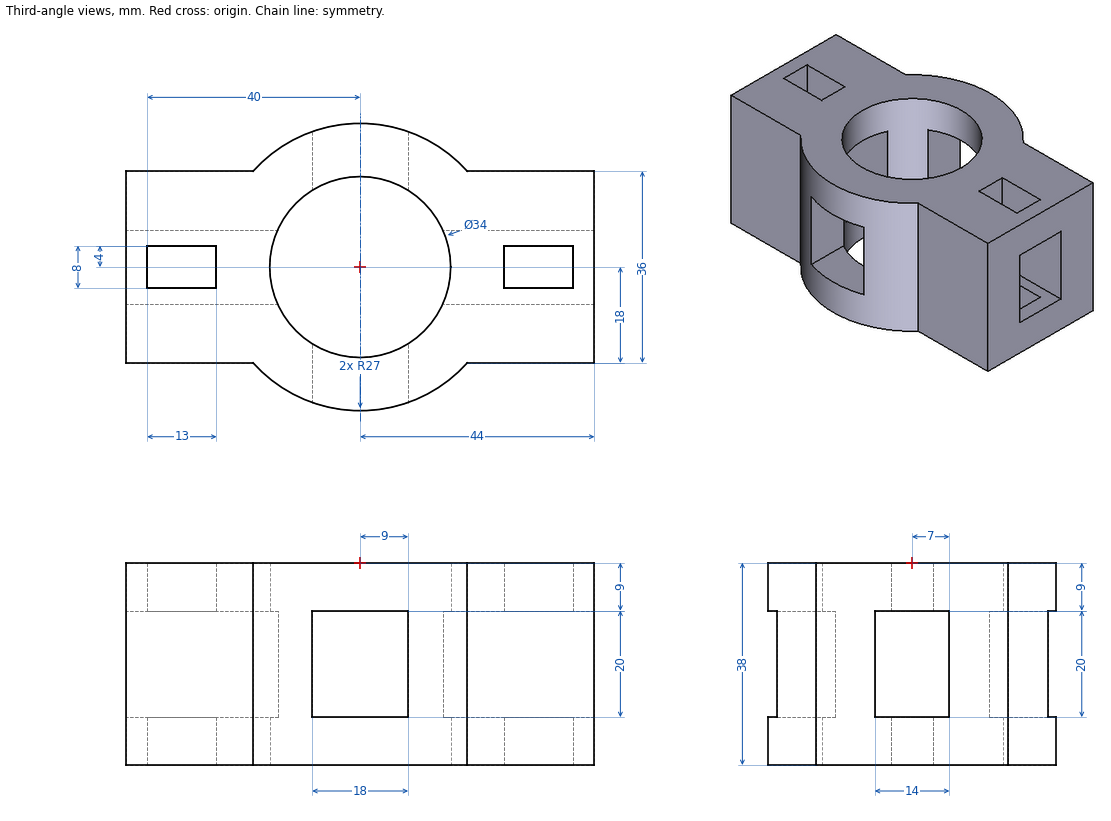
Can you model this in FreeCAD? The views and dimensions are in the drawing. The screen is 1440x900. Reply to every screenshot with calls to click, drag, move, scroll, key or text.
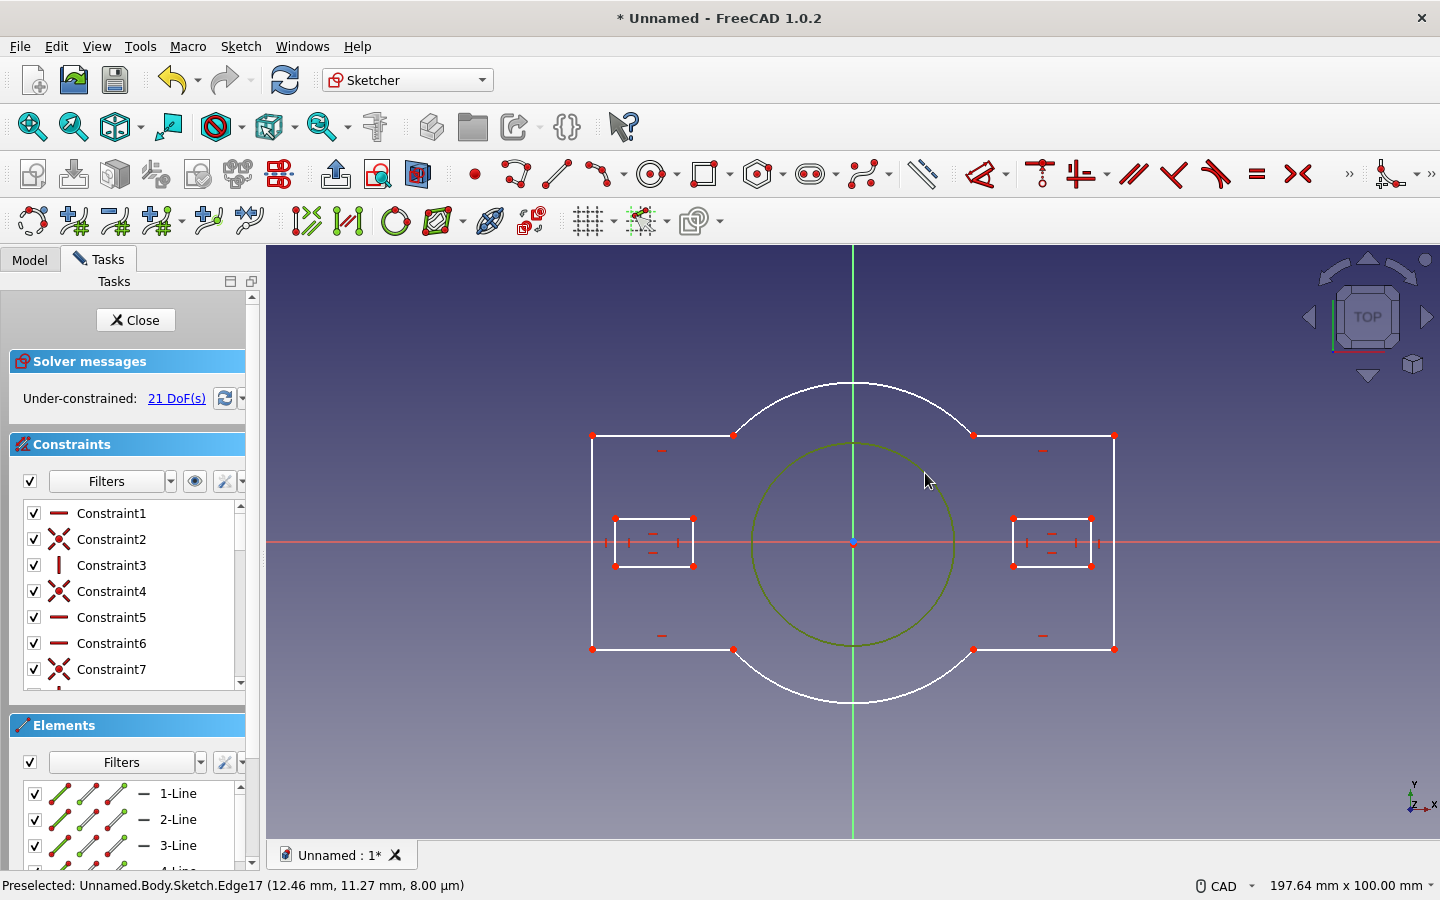
click(800, 694)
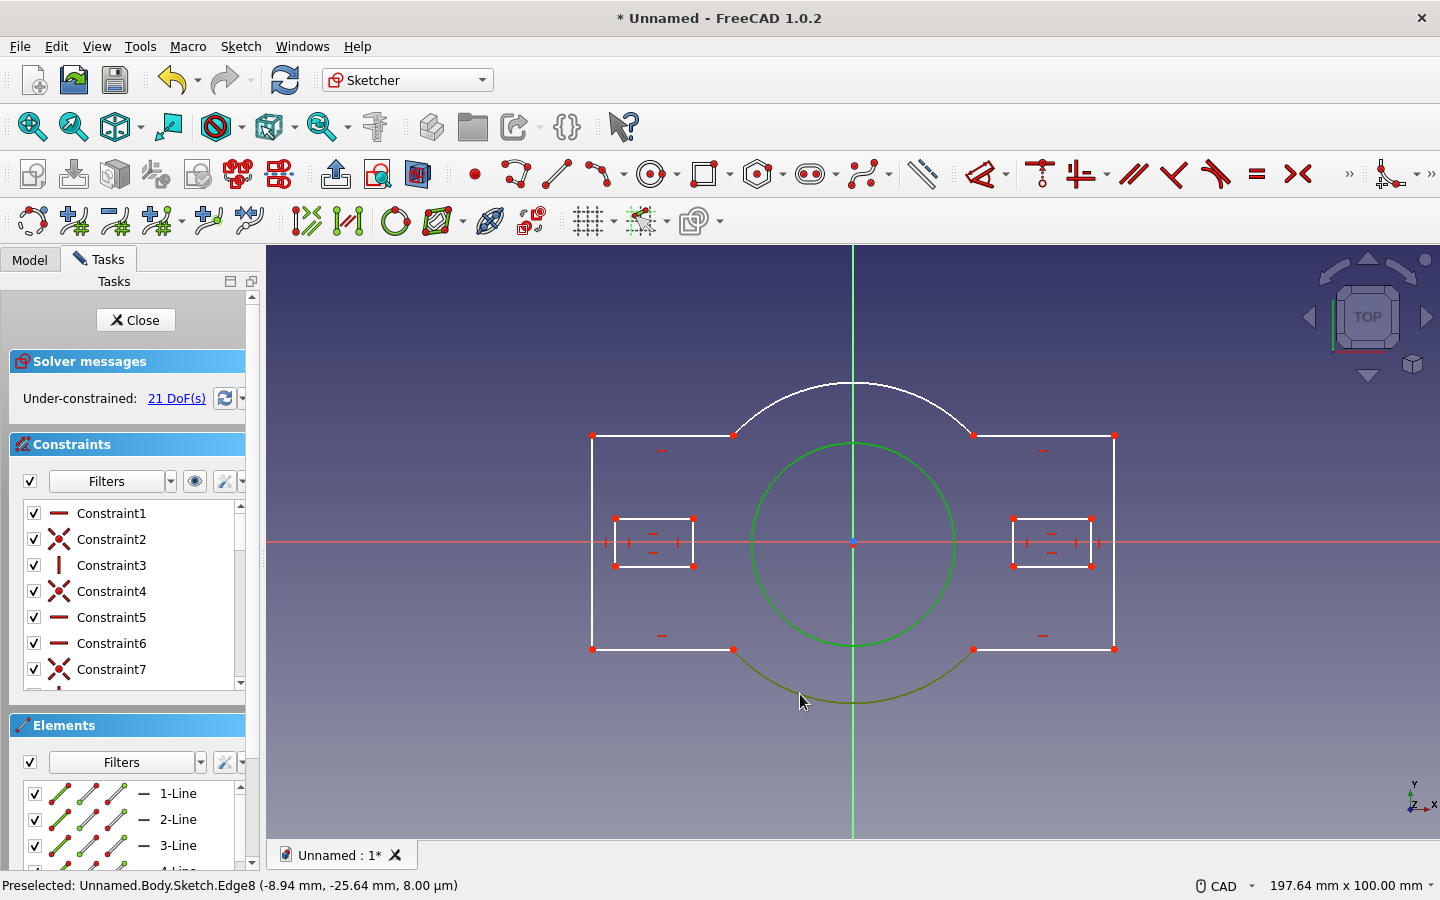
click(1040, 174)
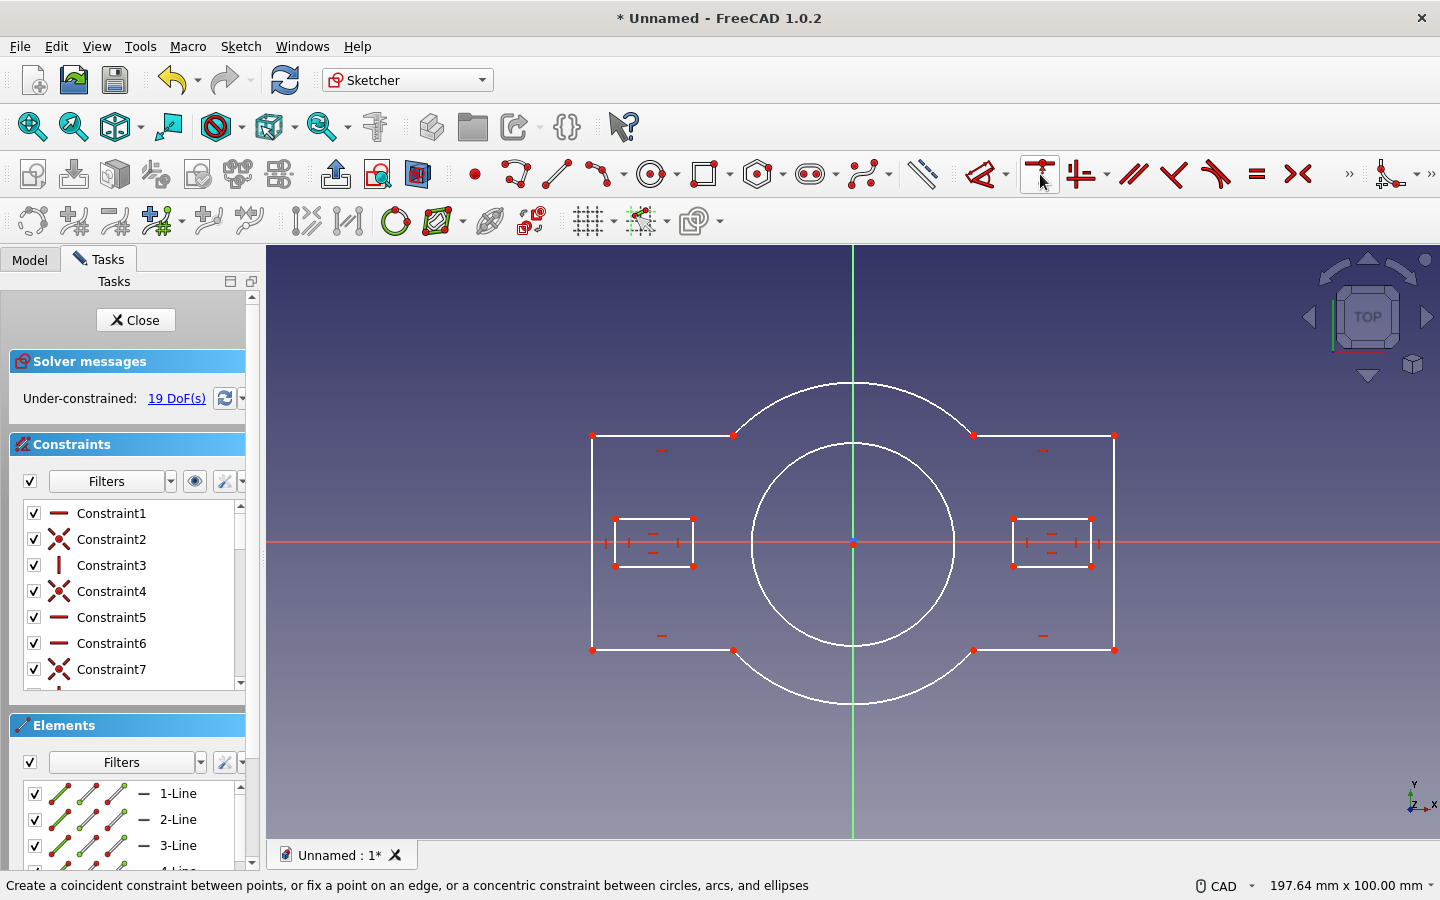
drag(843, 532, 863, 555)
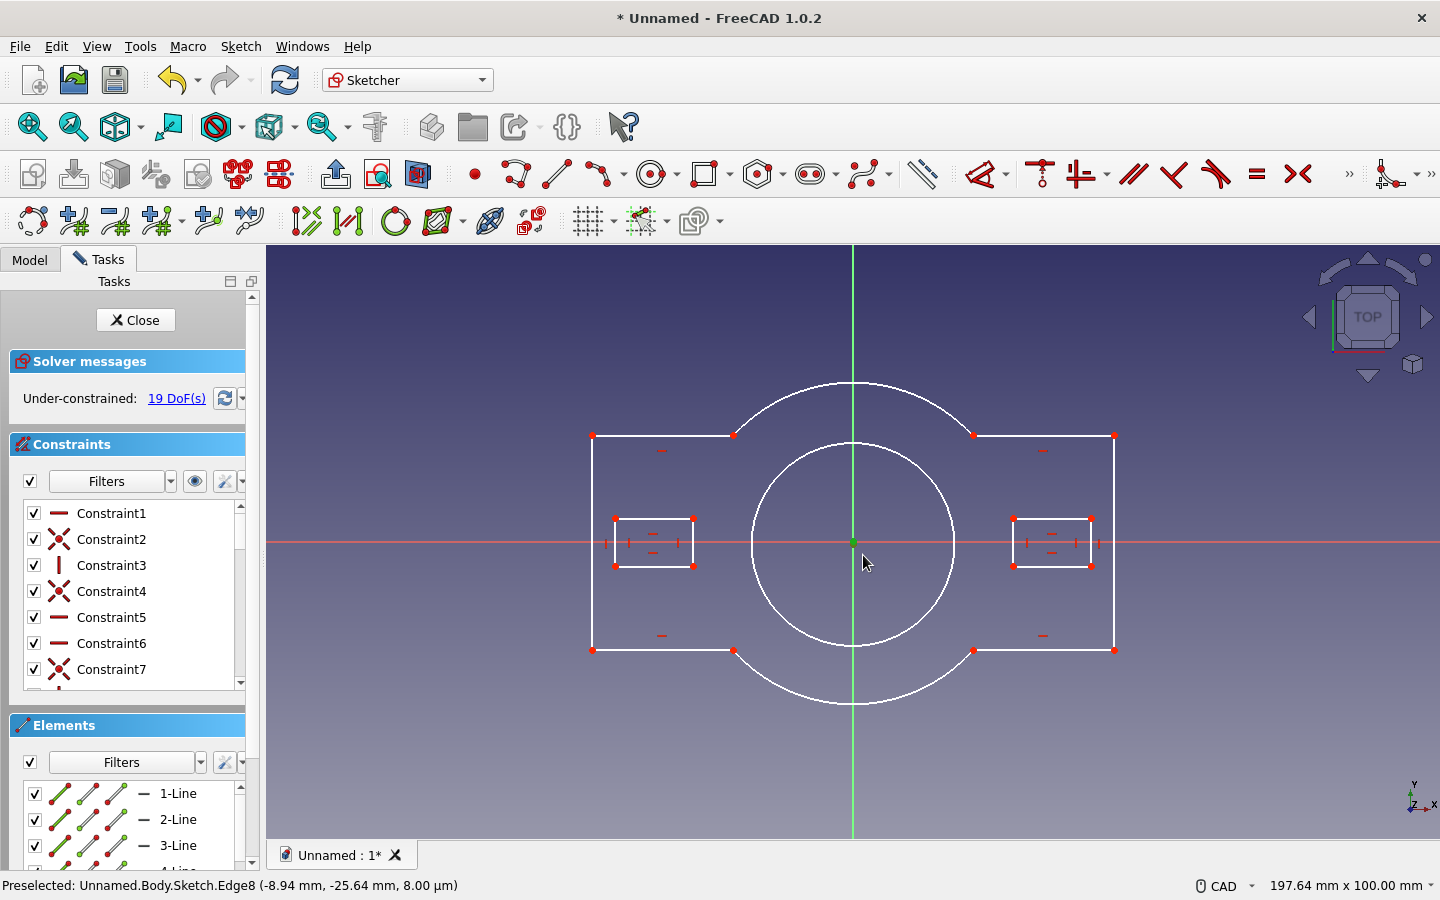
key(c)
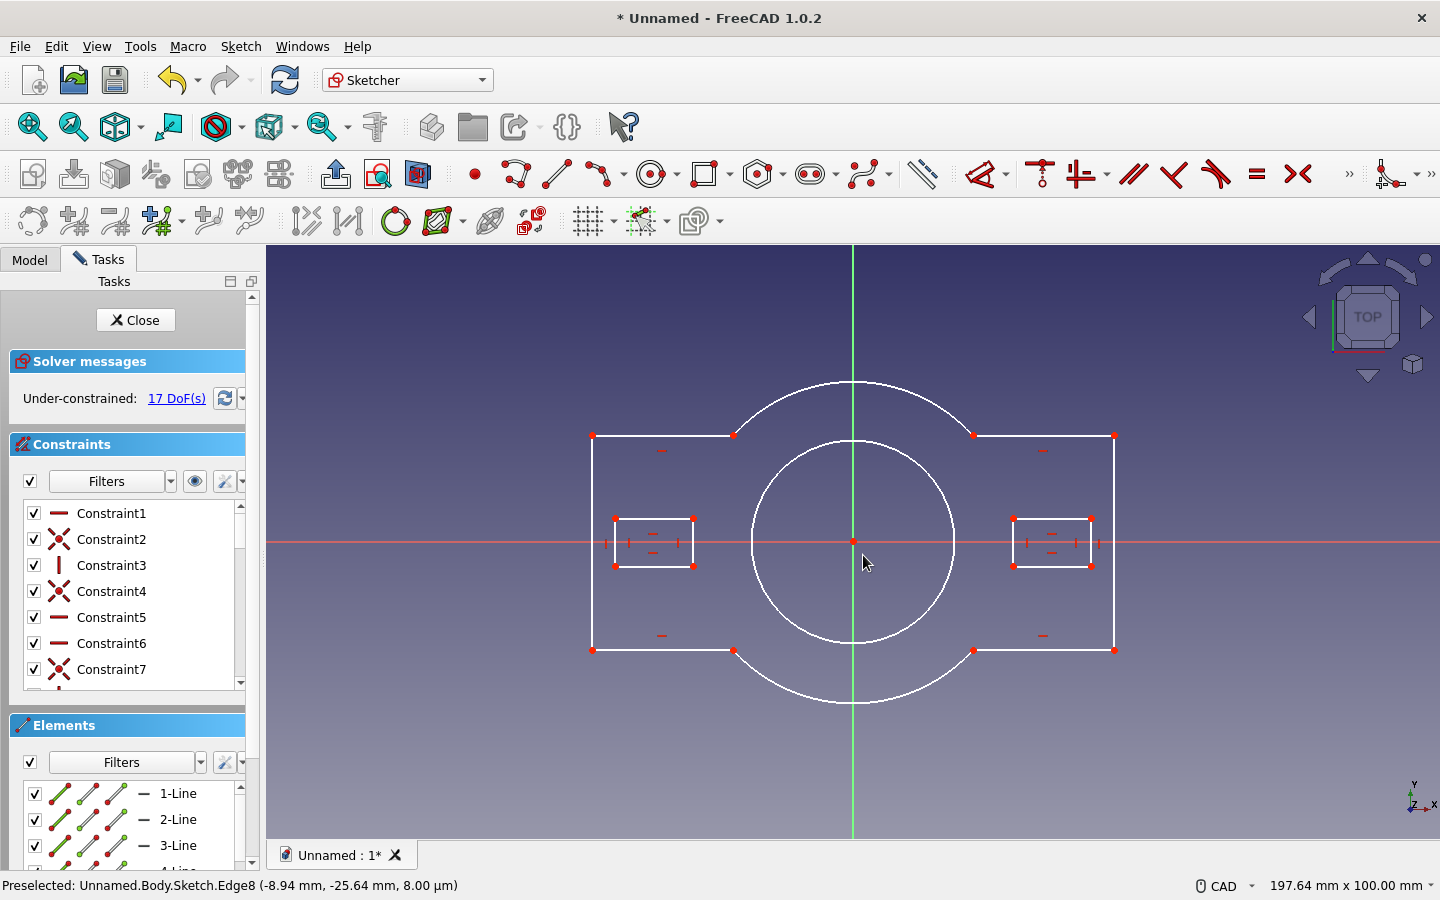
click(906, 391)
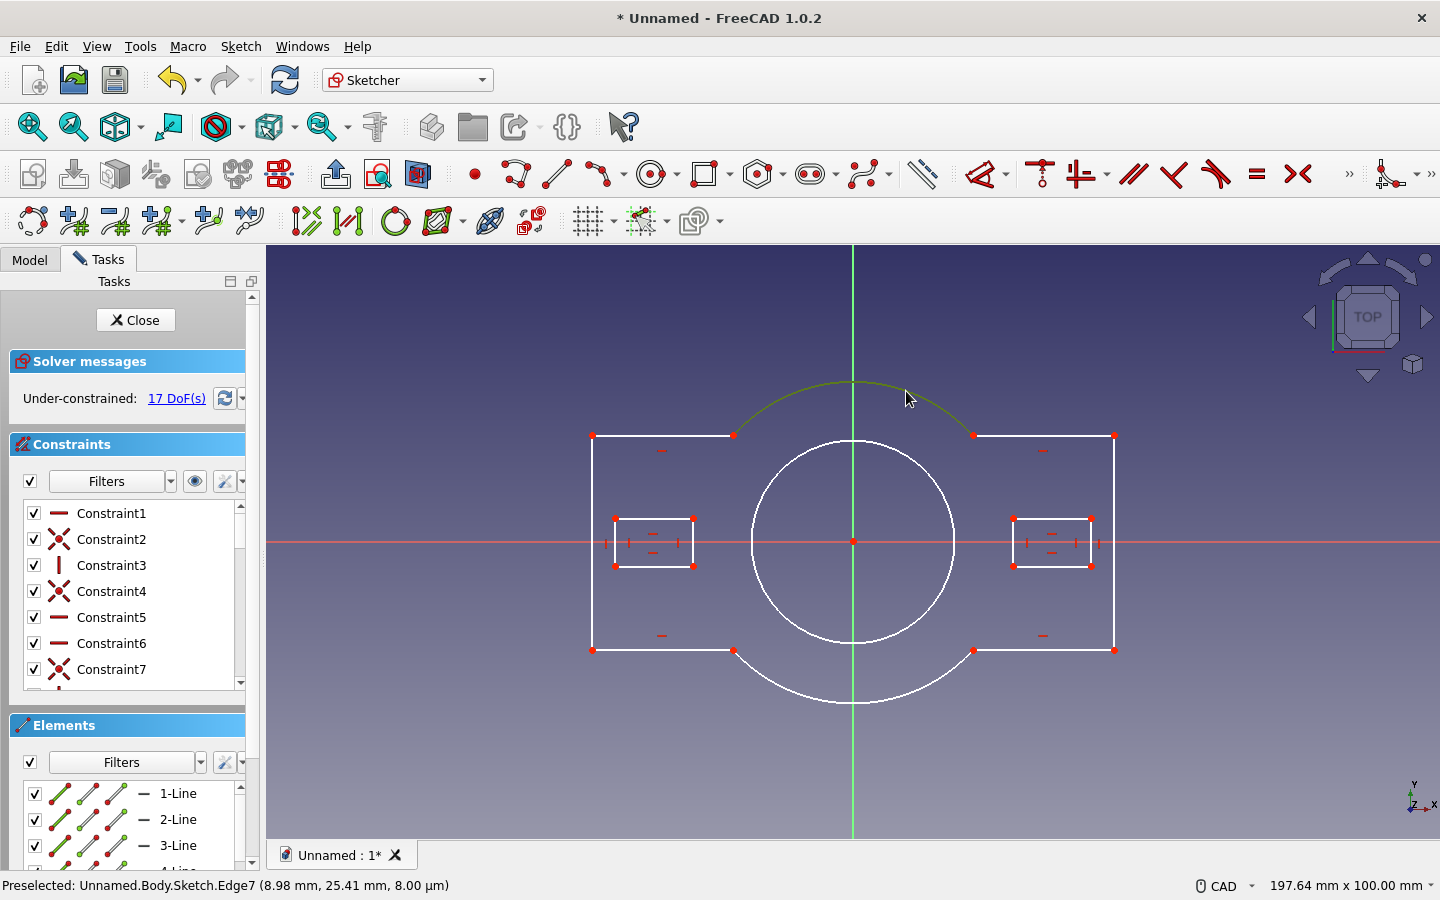
click(800, 694)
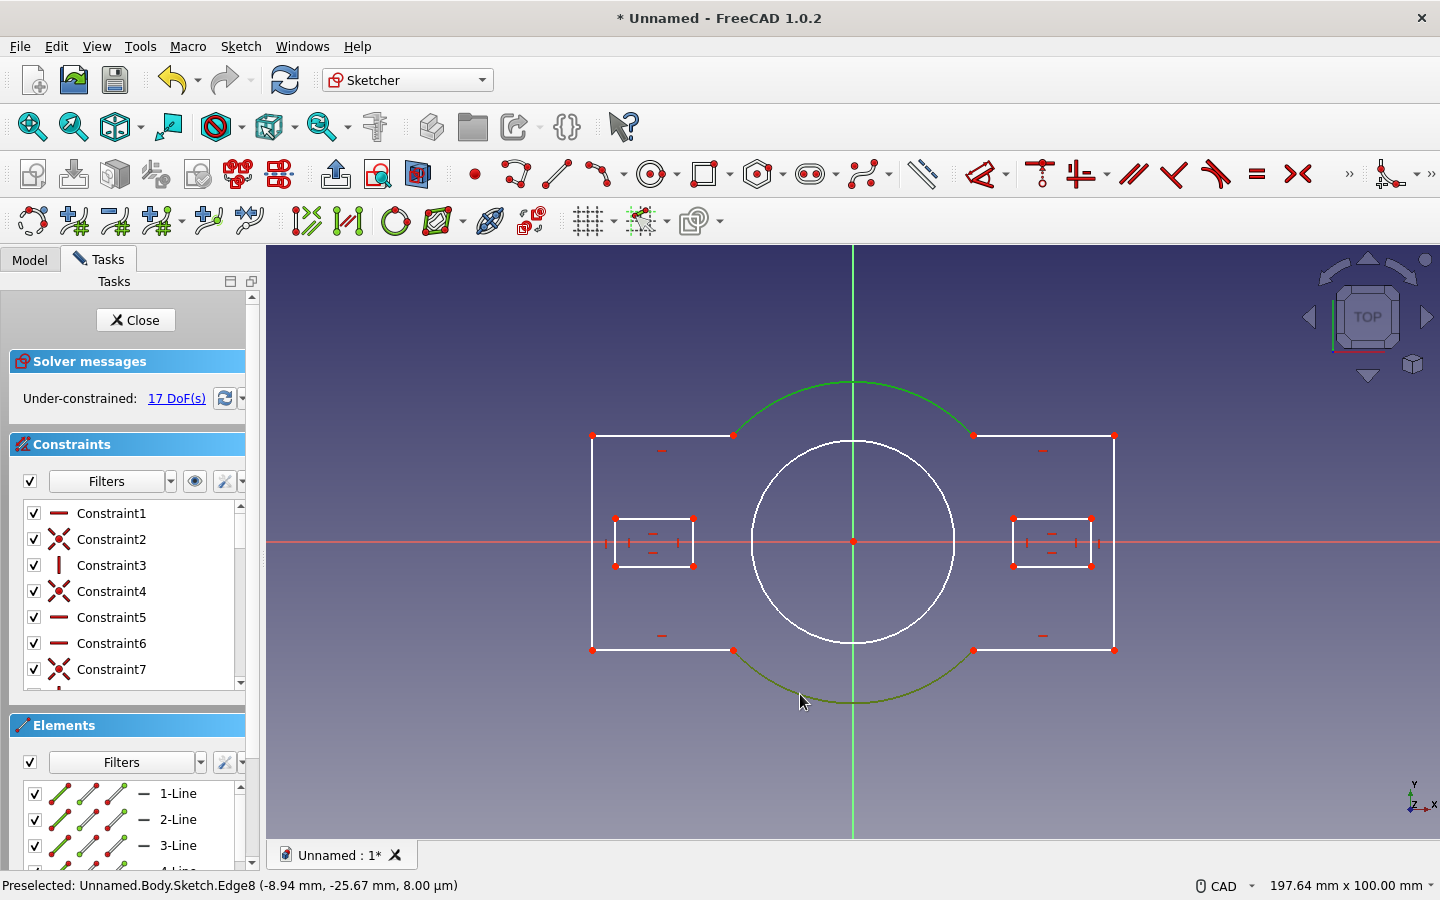
click(1257, 174)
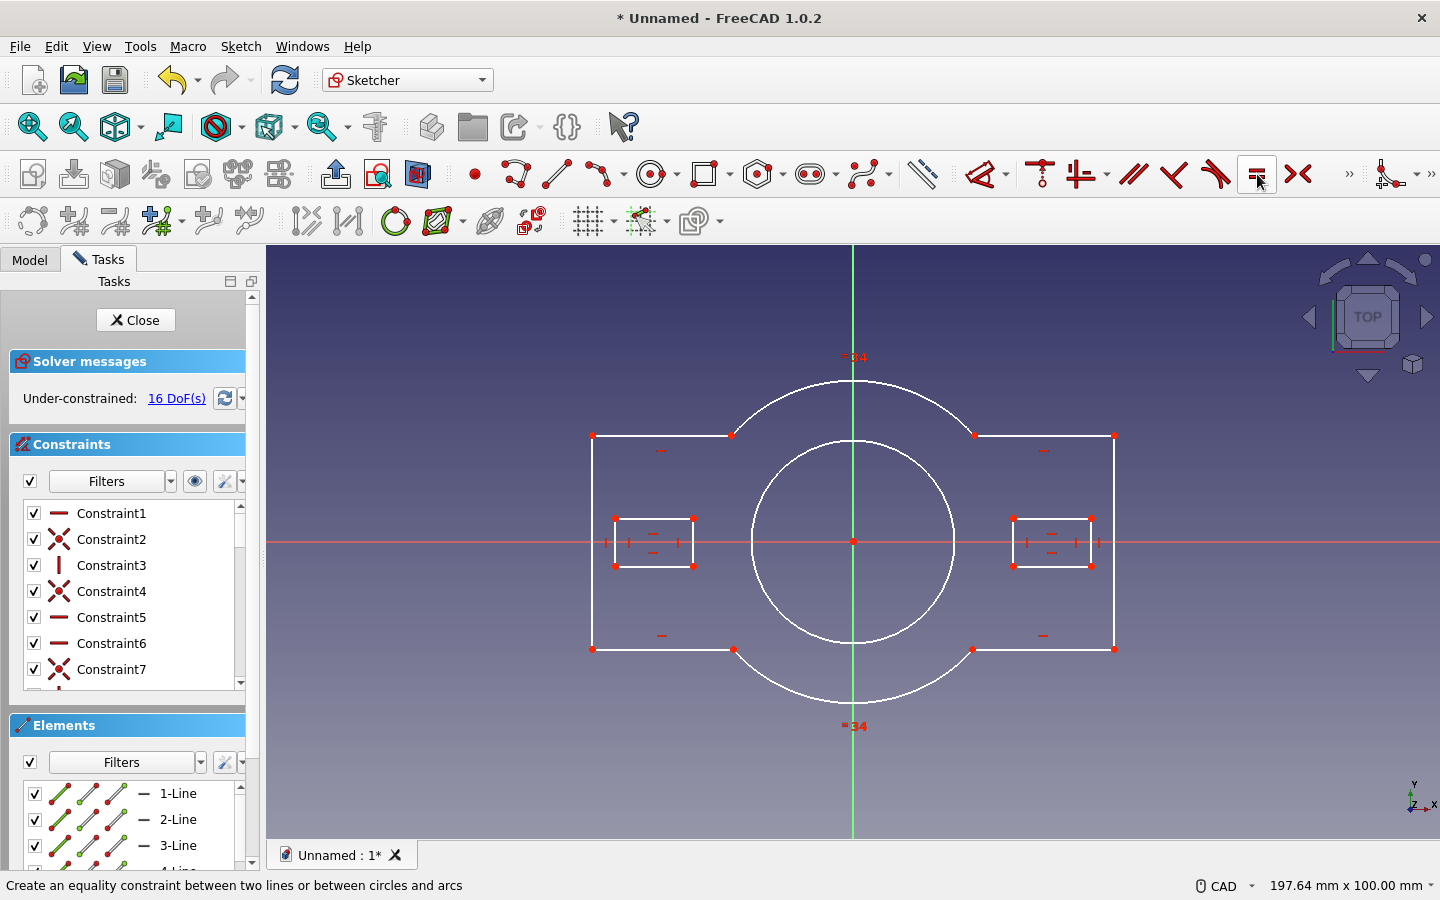
click(1114, 436)